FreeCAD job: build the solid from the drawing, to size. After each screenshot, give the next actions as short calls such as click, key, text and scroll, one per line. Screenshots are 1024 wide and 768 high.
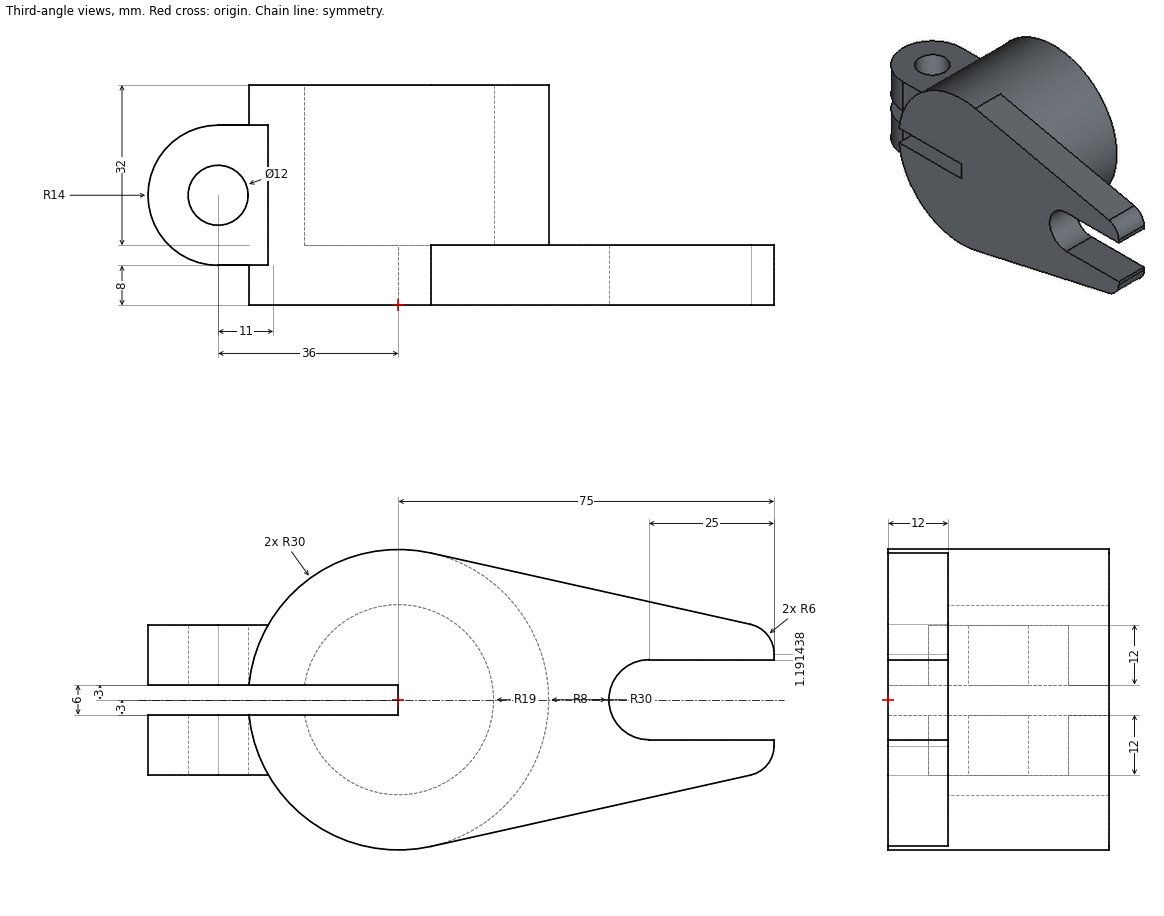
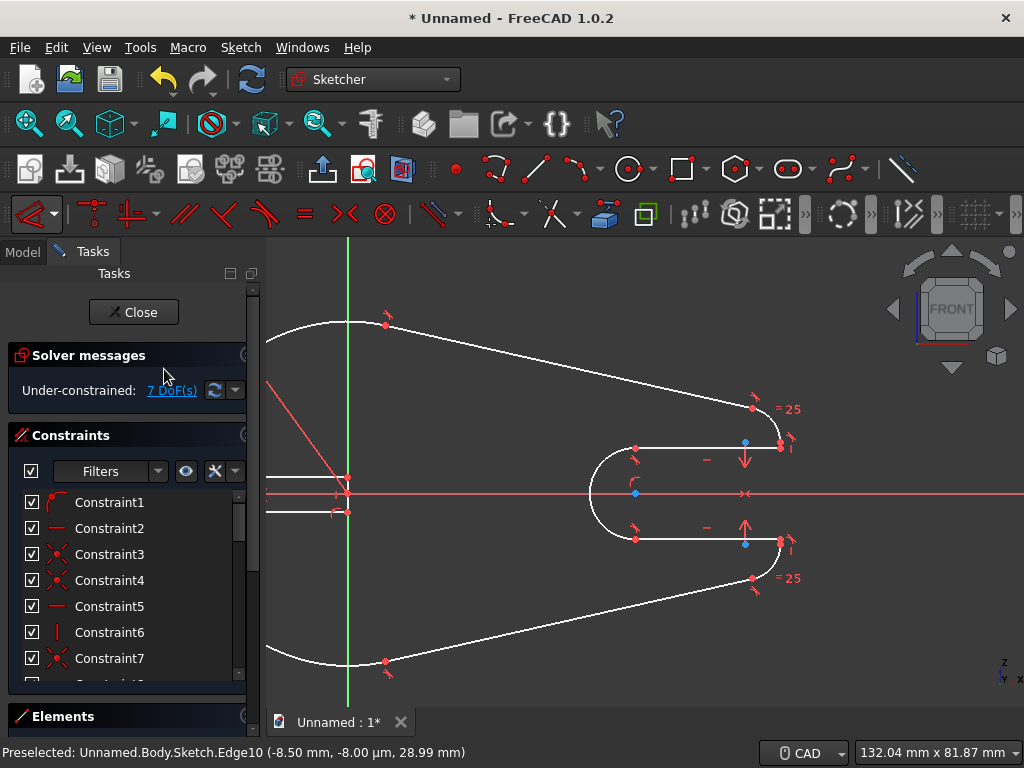
click(777, 429)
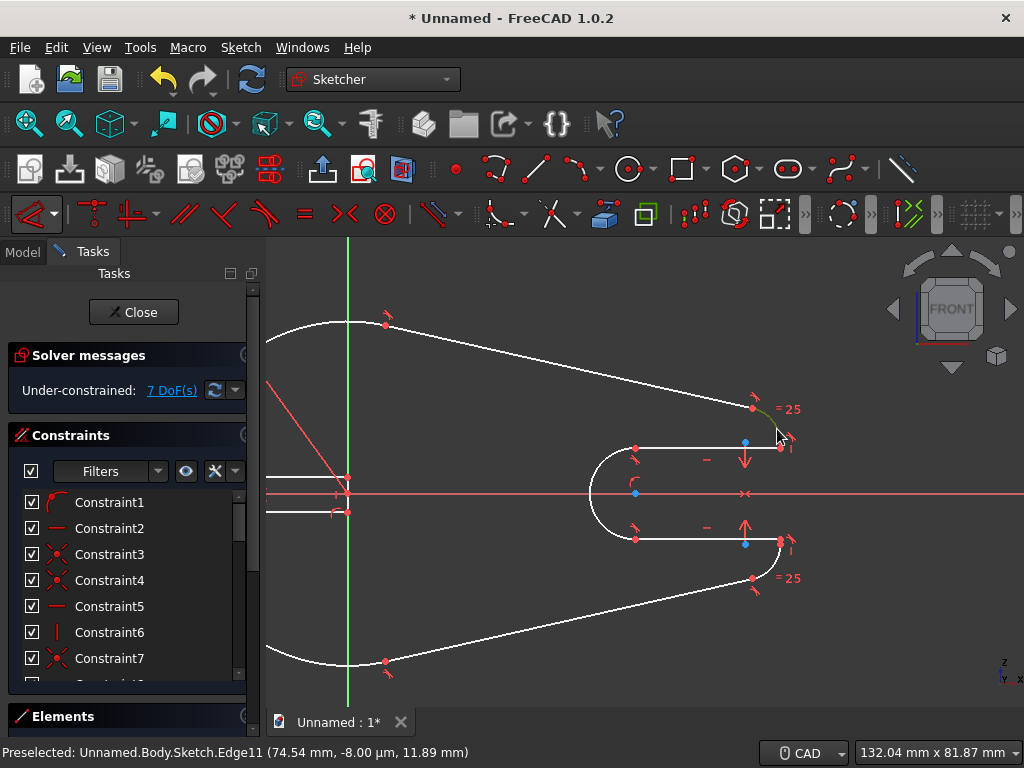
key(k)
key(r)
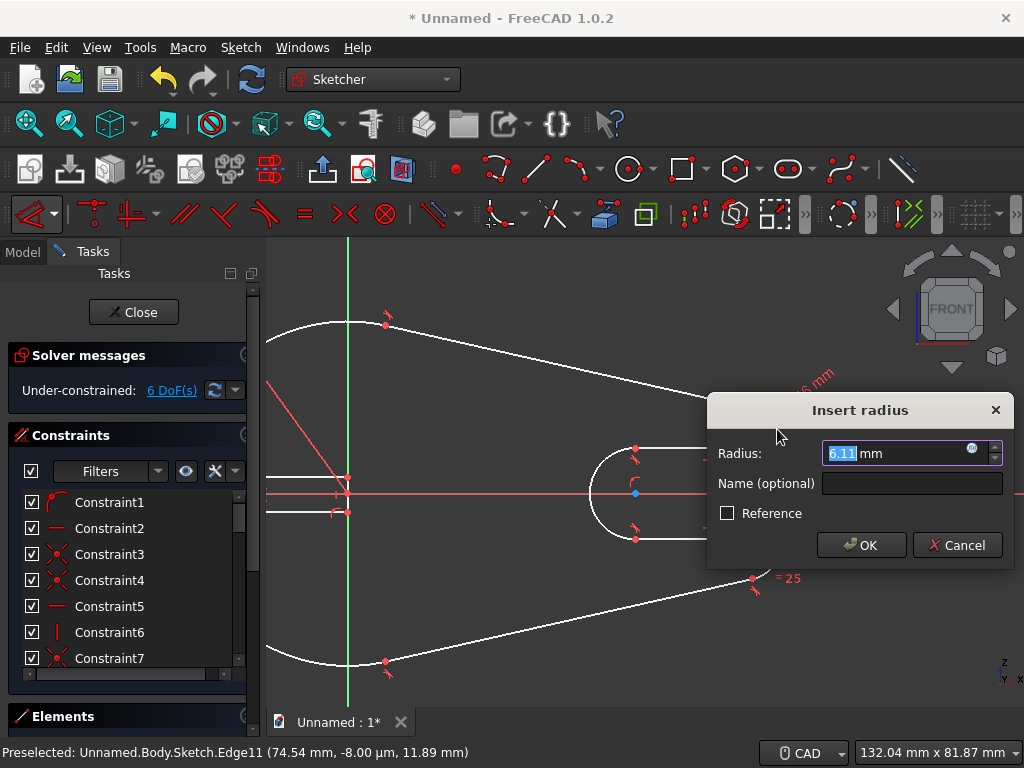
text(6)
key(Return)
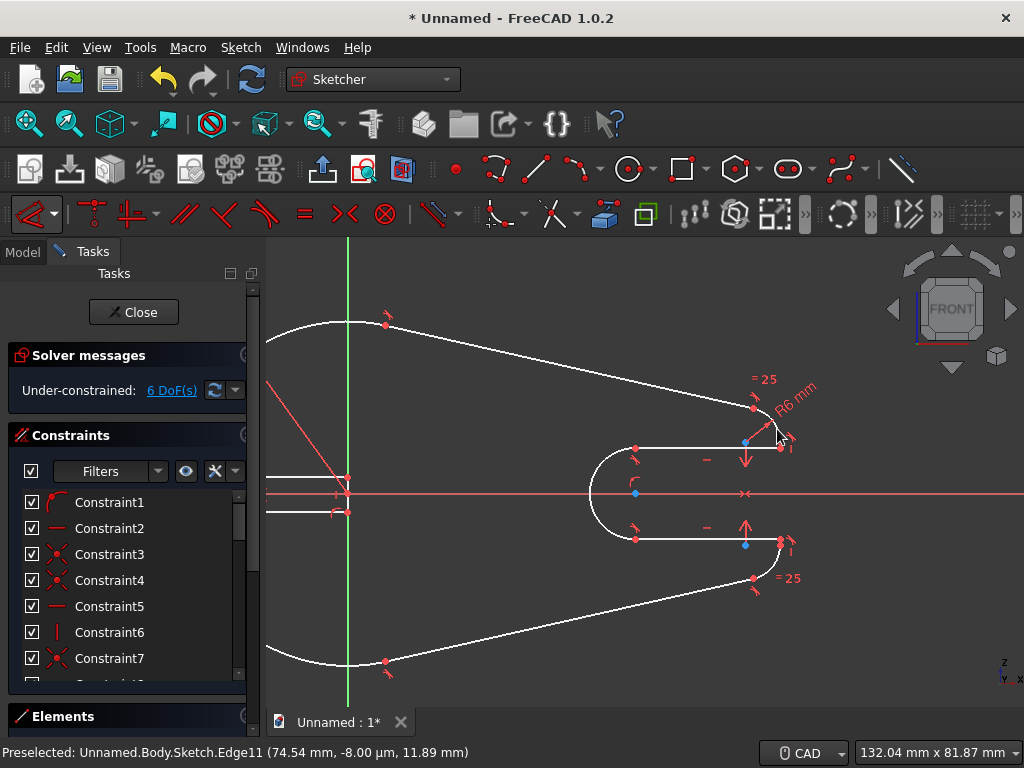
click(599, 467)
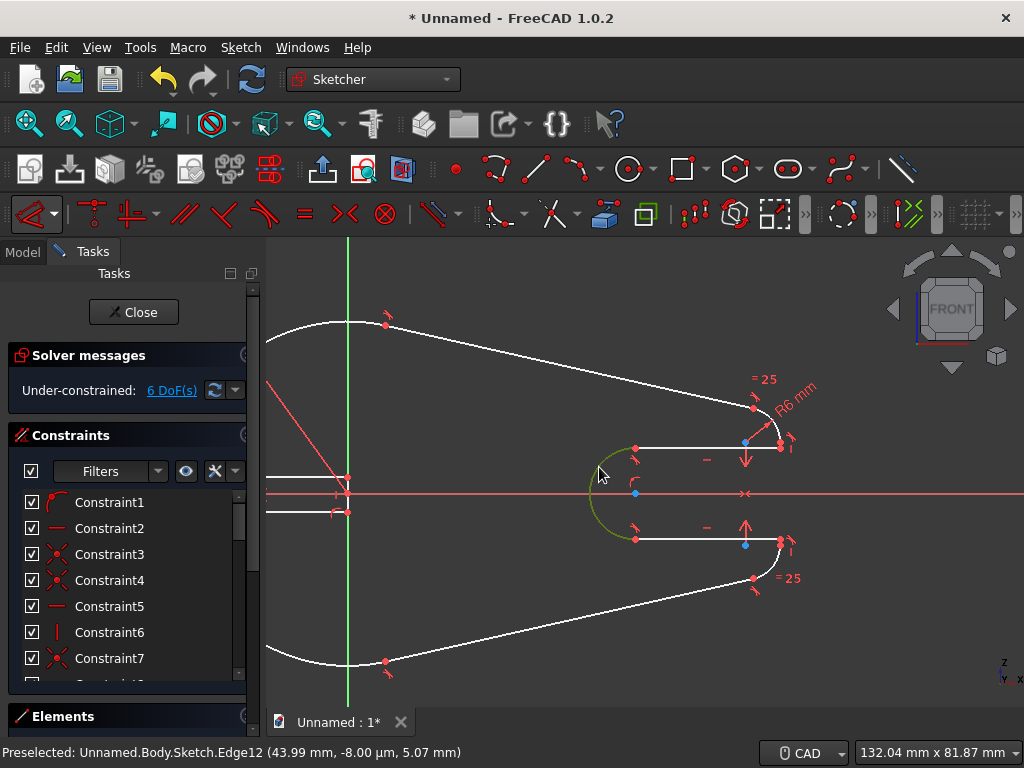
key(k)
key(r)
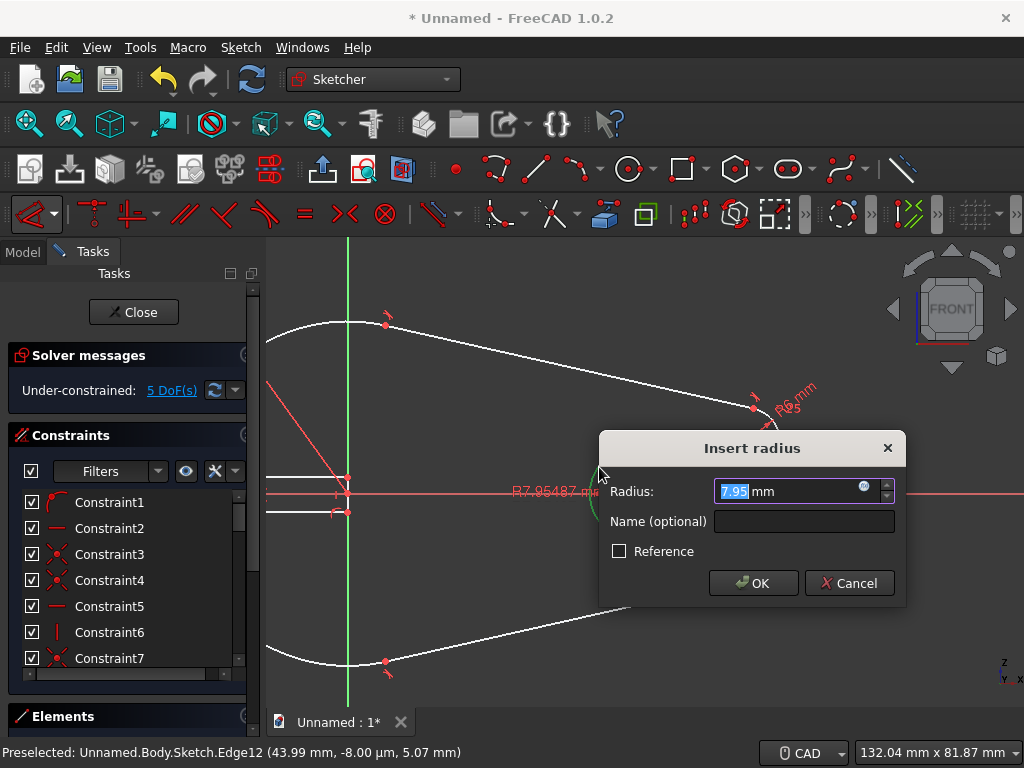
text(8)
key(Return)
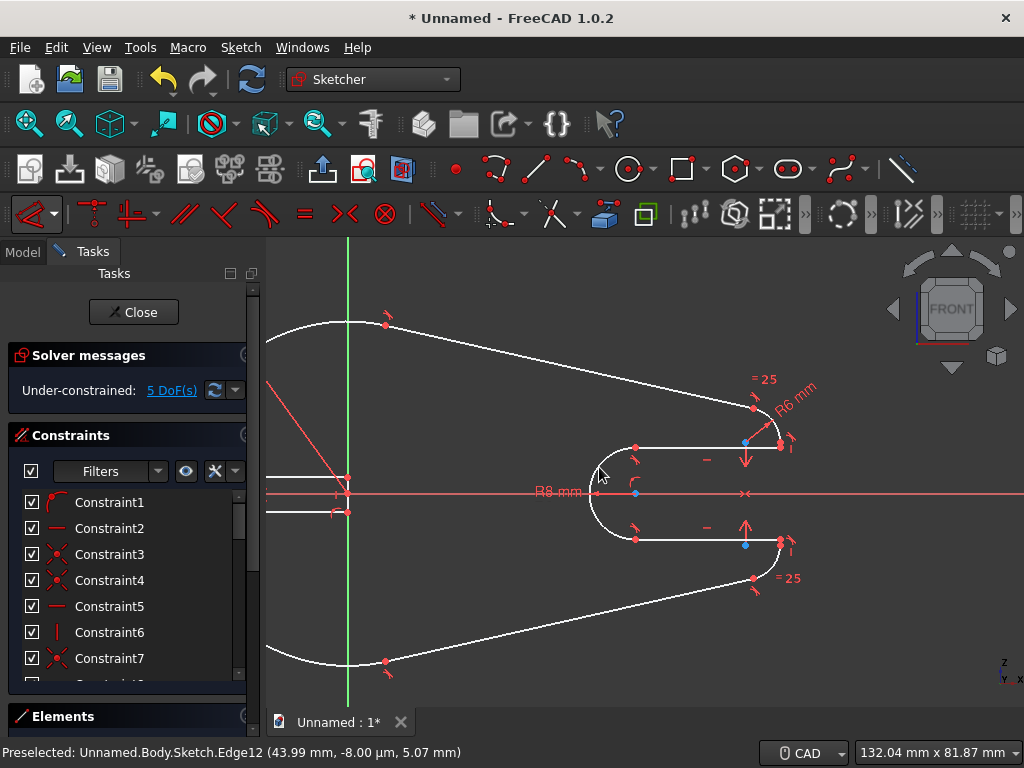
click(348, 502)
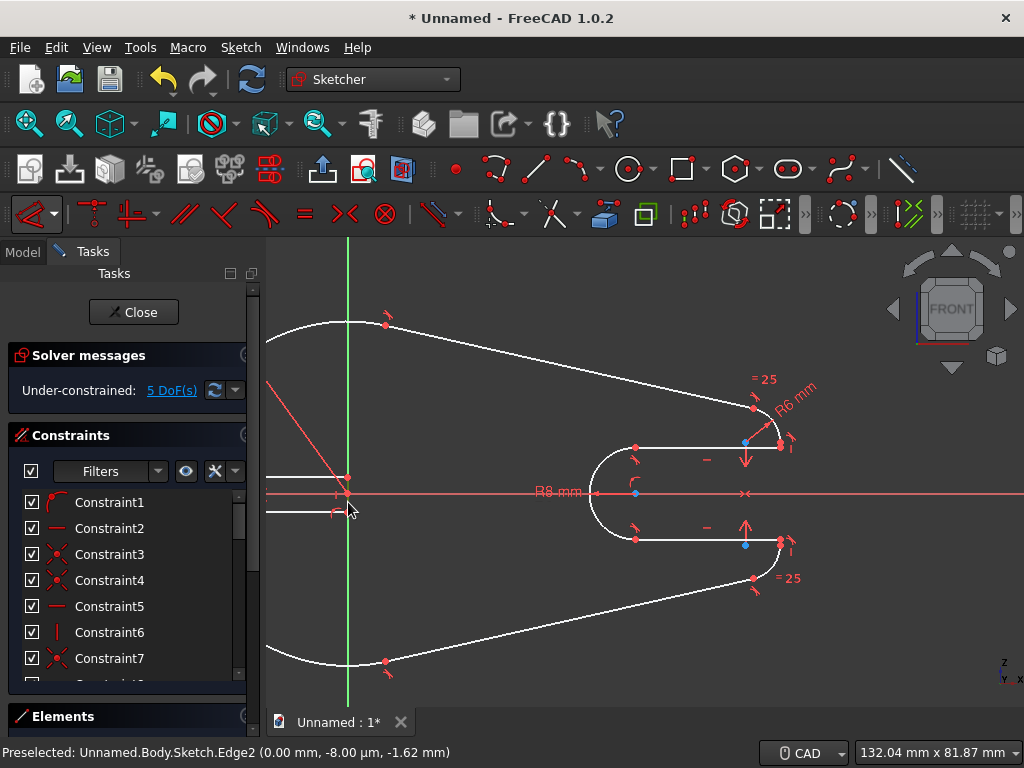
key(i)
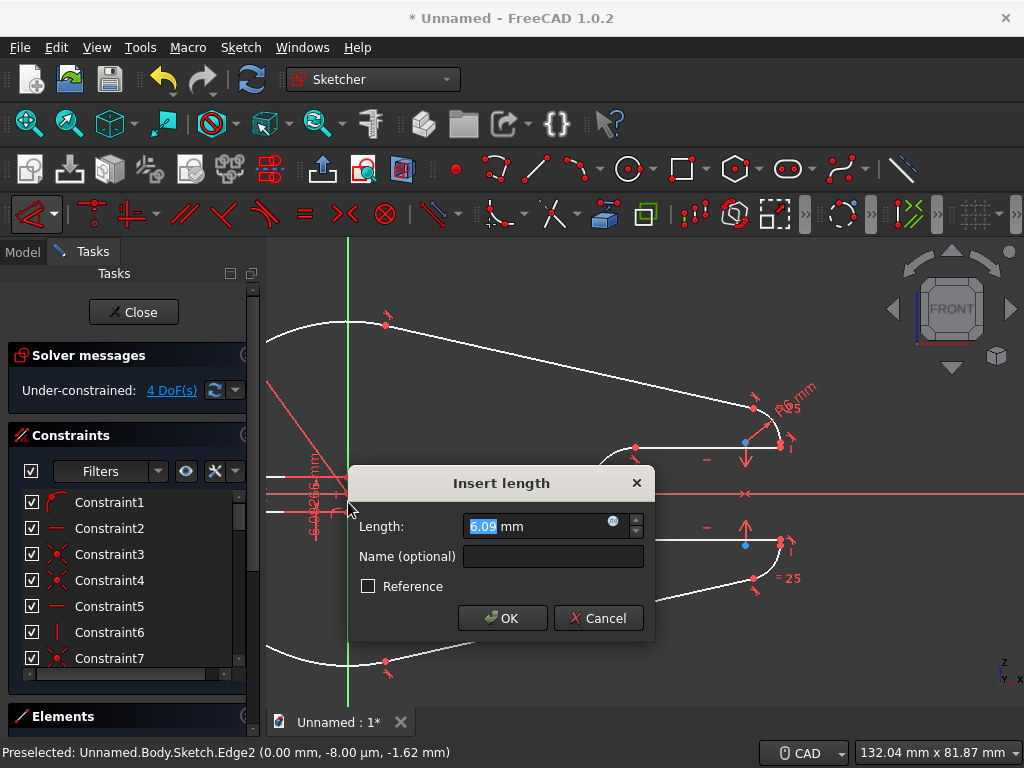
text(6)
key(Return)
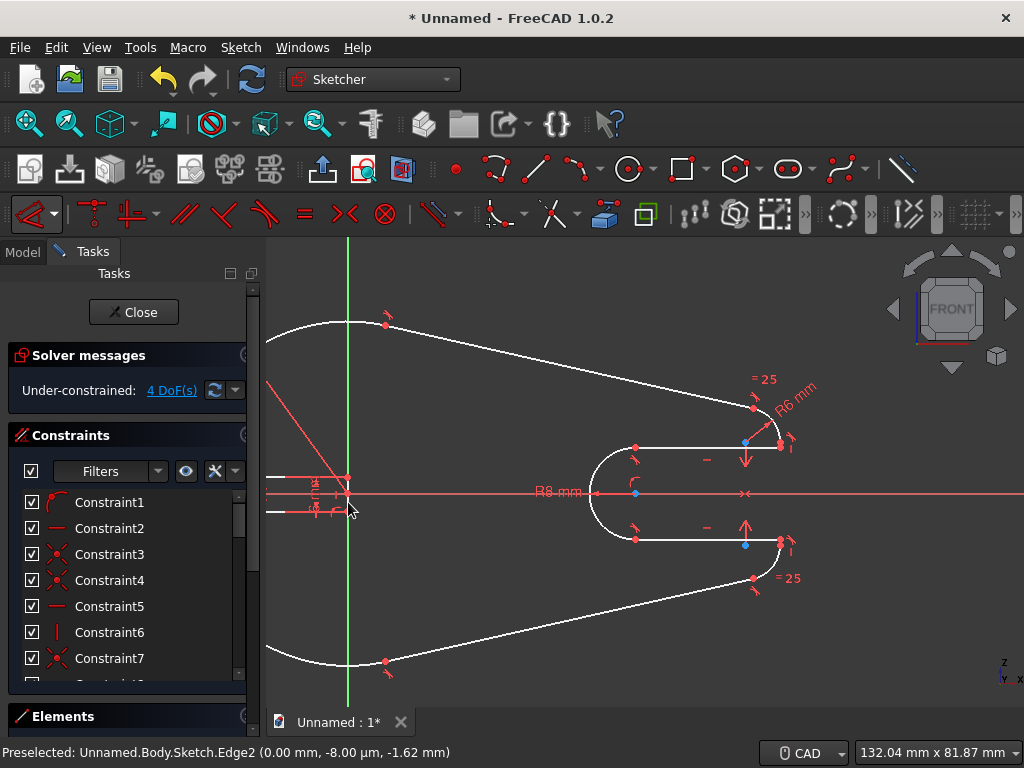
click(737, 448)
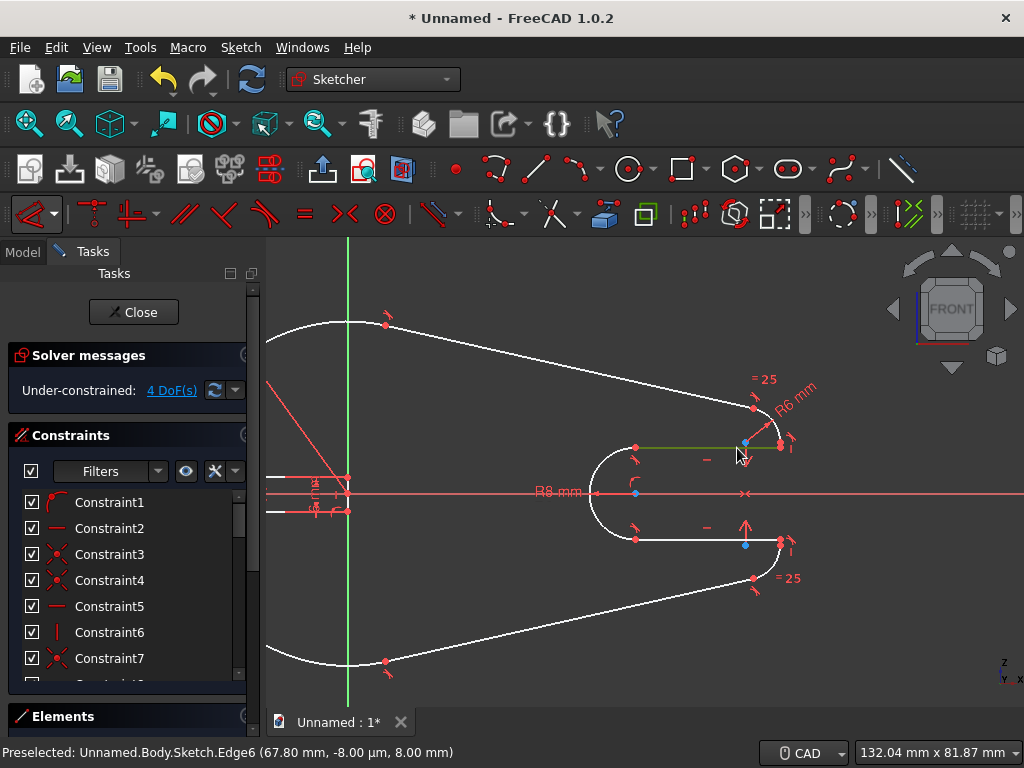
key(l)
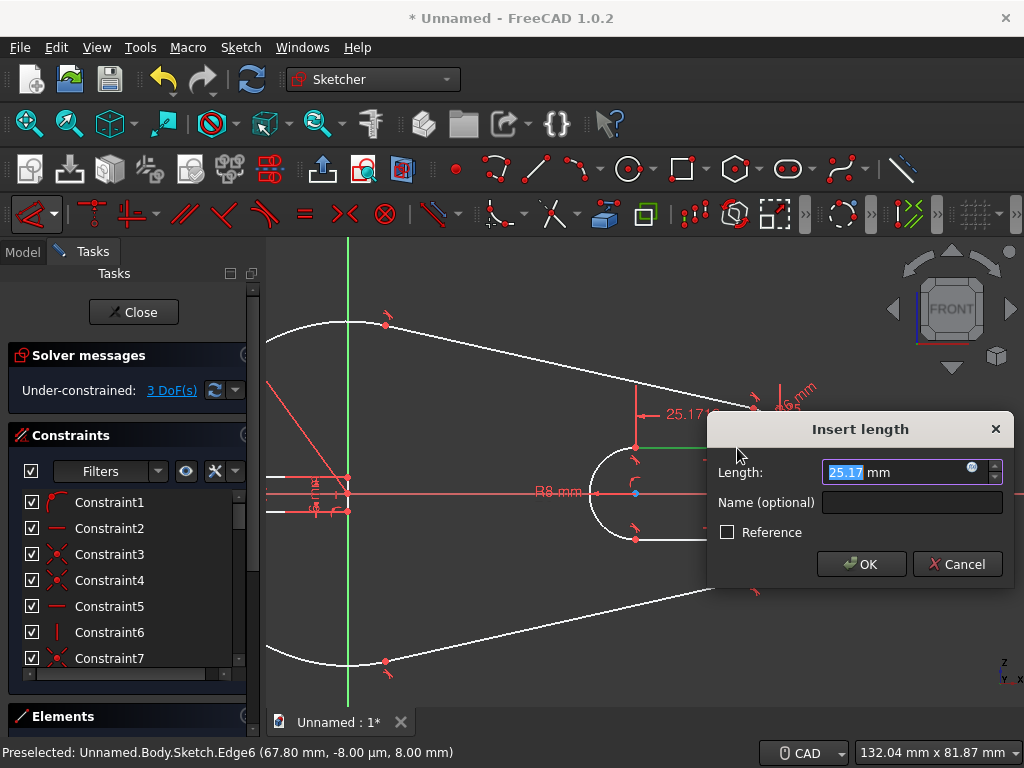
text(25)
key(Return)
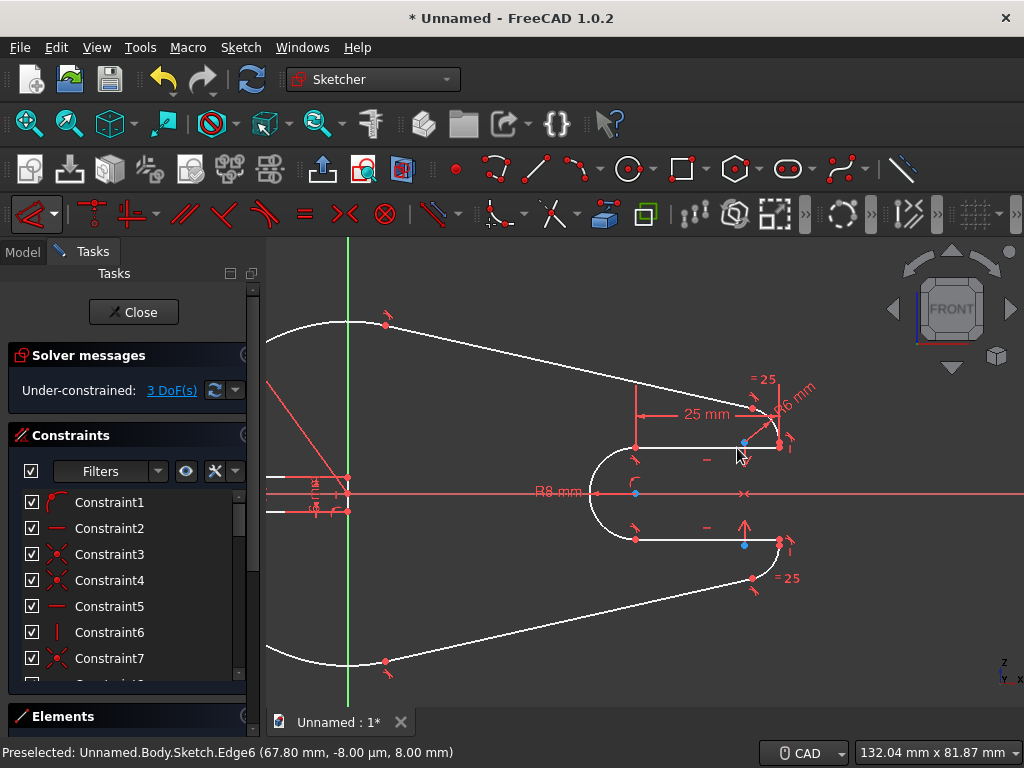
scroll(778, 428, down, 2)